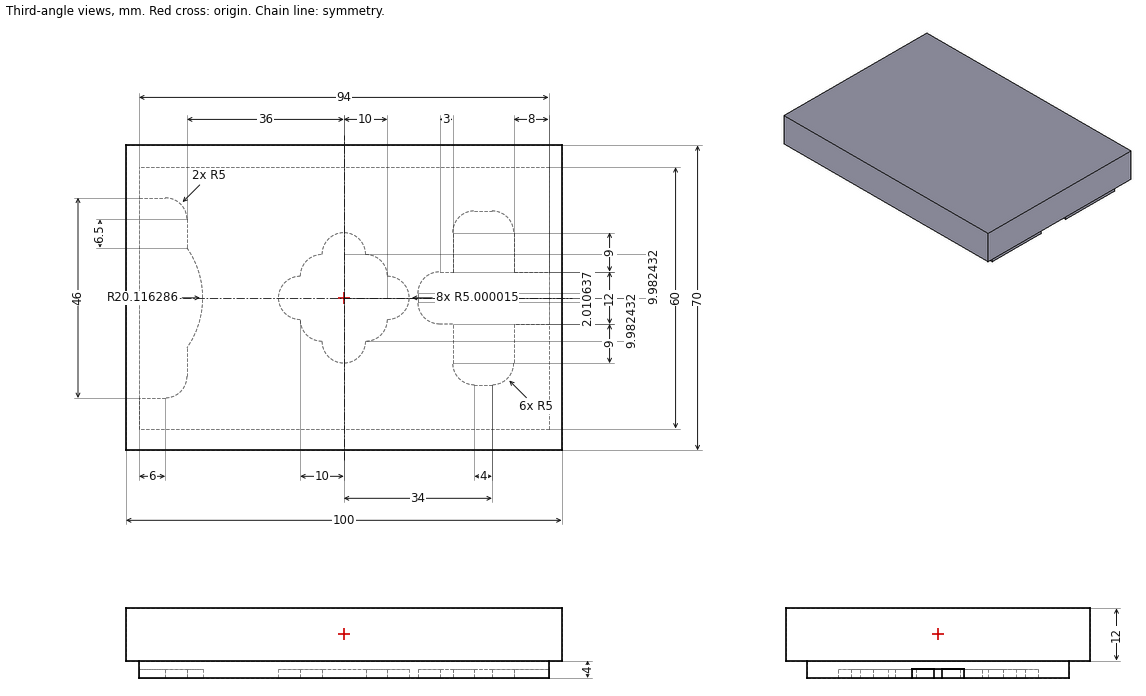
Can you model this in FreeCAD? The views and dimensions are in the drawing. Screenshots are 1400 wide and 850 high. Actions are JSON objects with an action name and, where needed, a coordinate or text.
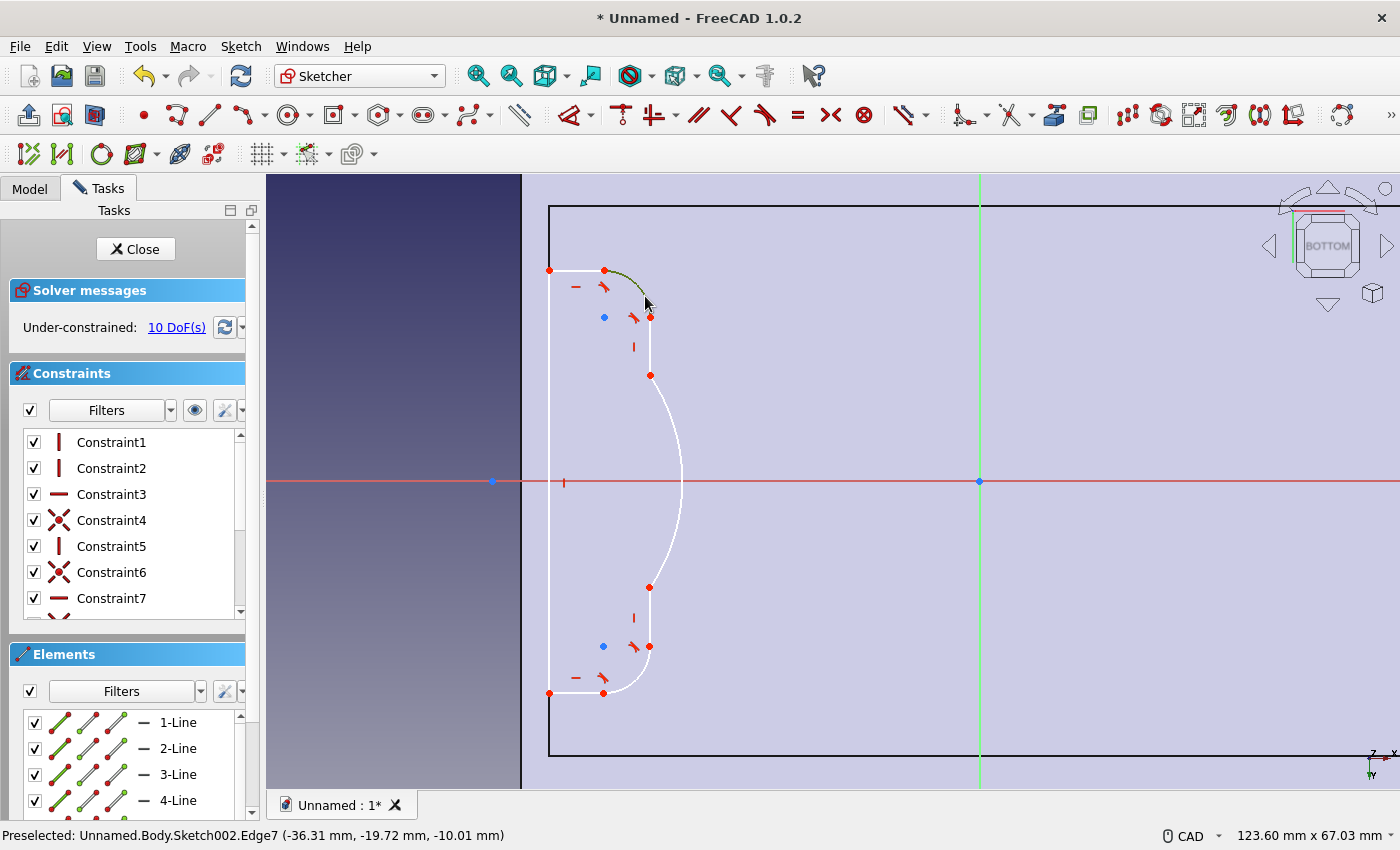
{"action": "left_click", "coordinate": [625, 688]}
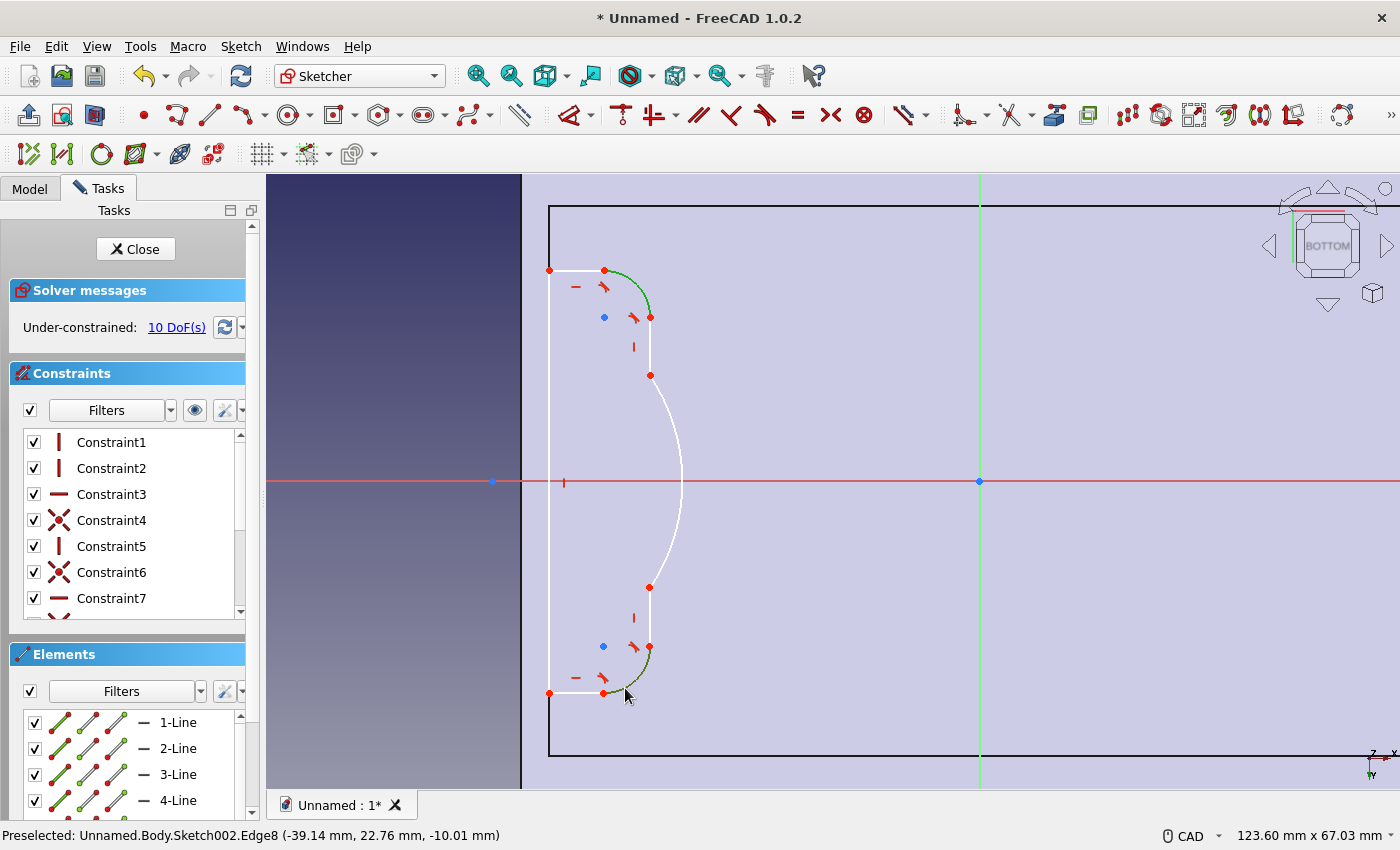
{"action": "left_click", "coordinate": [798, 116]}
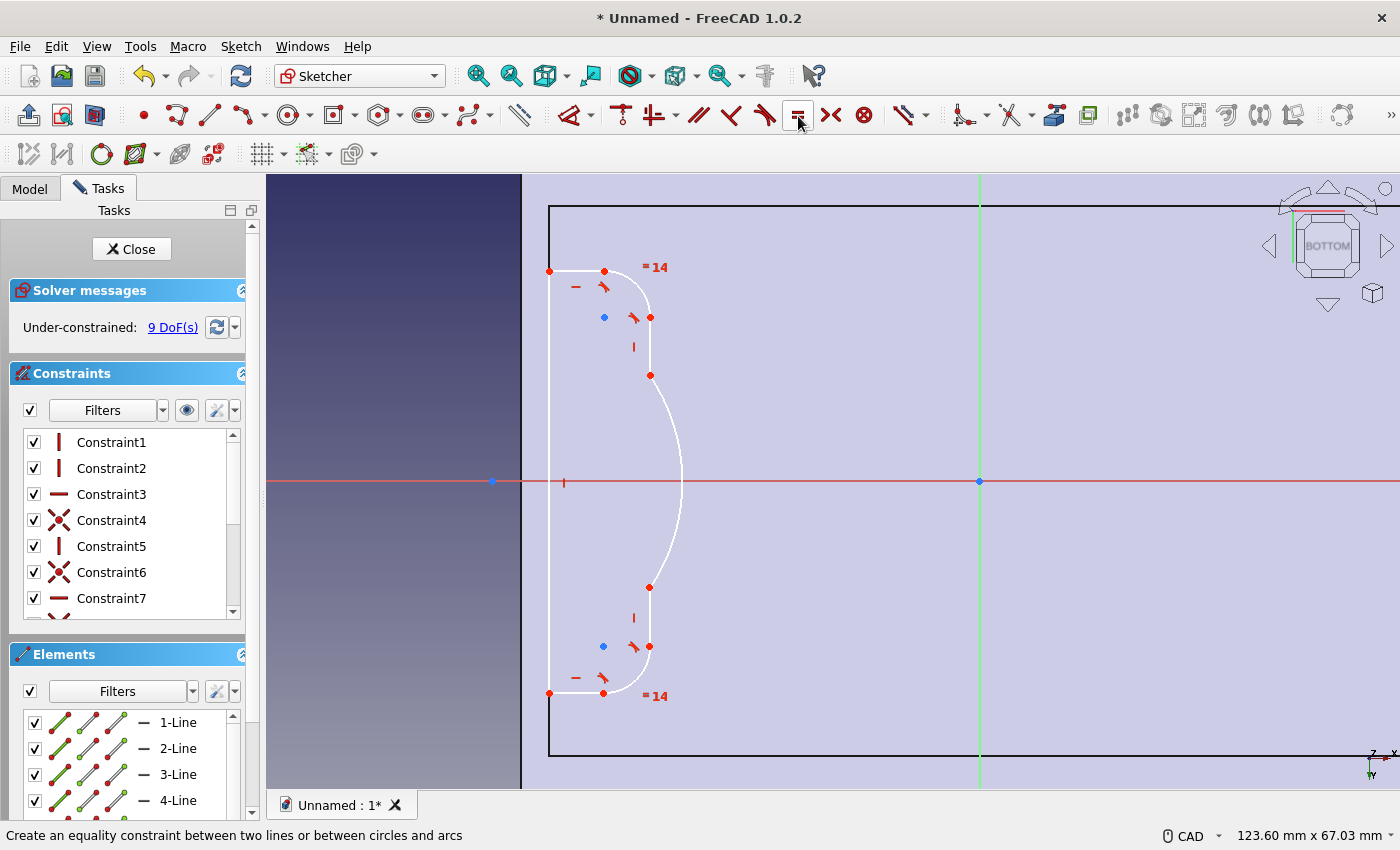
{"action": "left_click", "coordinate": [492, 482]}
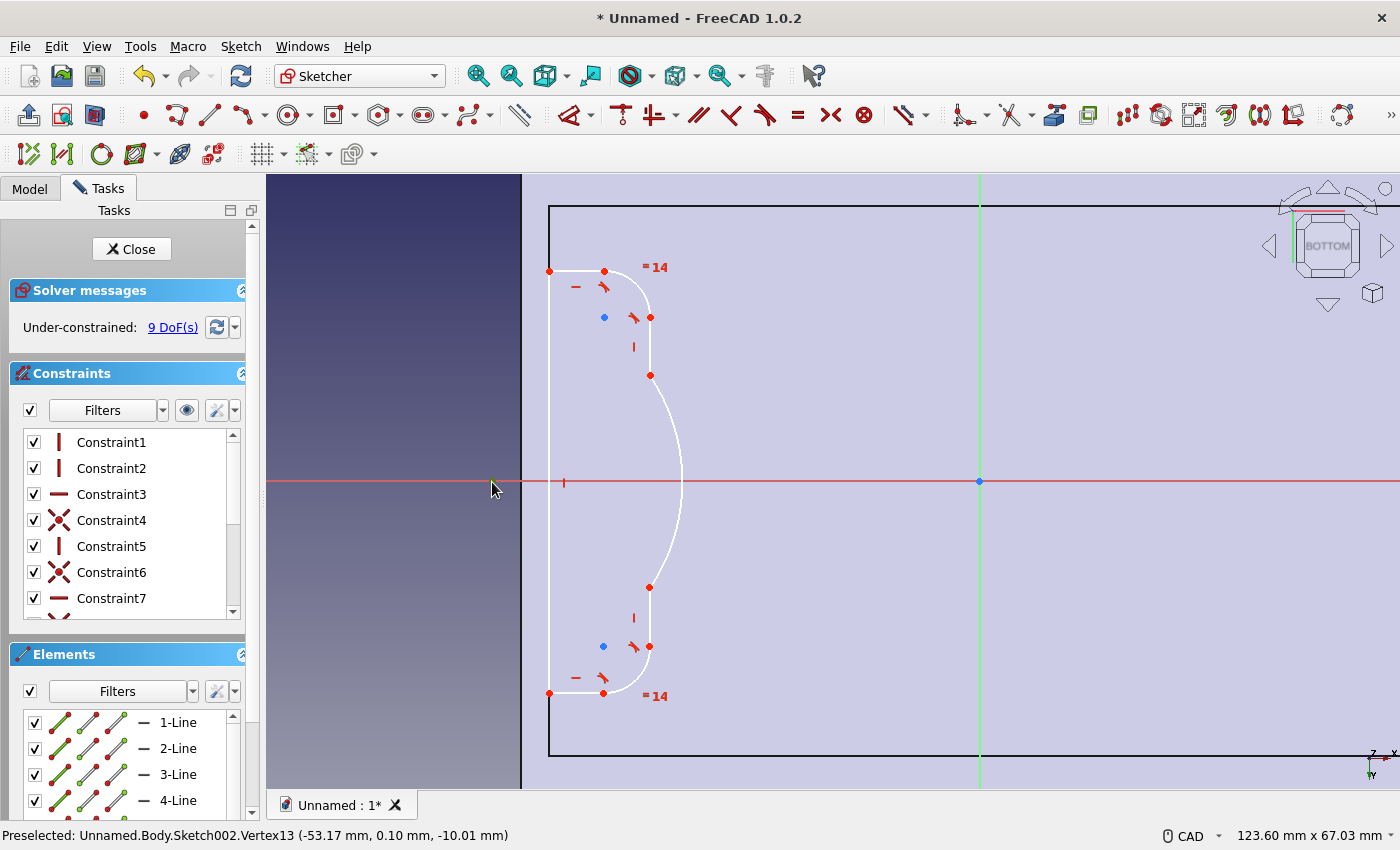
{"action": "left_click", "coordinate": [361, 481]}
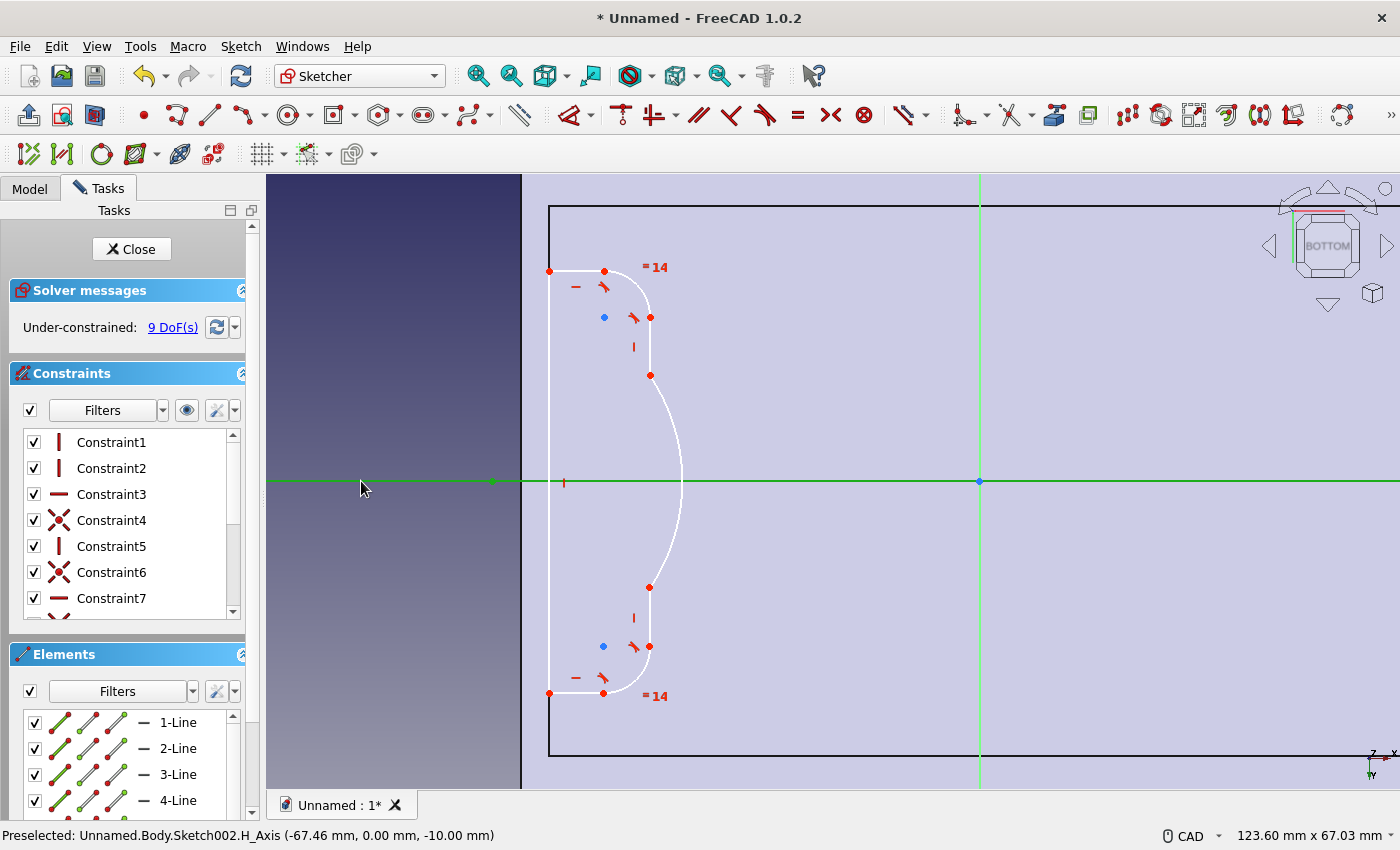
{"action": "left_click", "coordinate": [621, 116]}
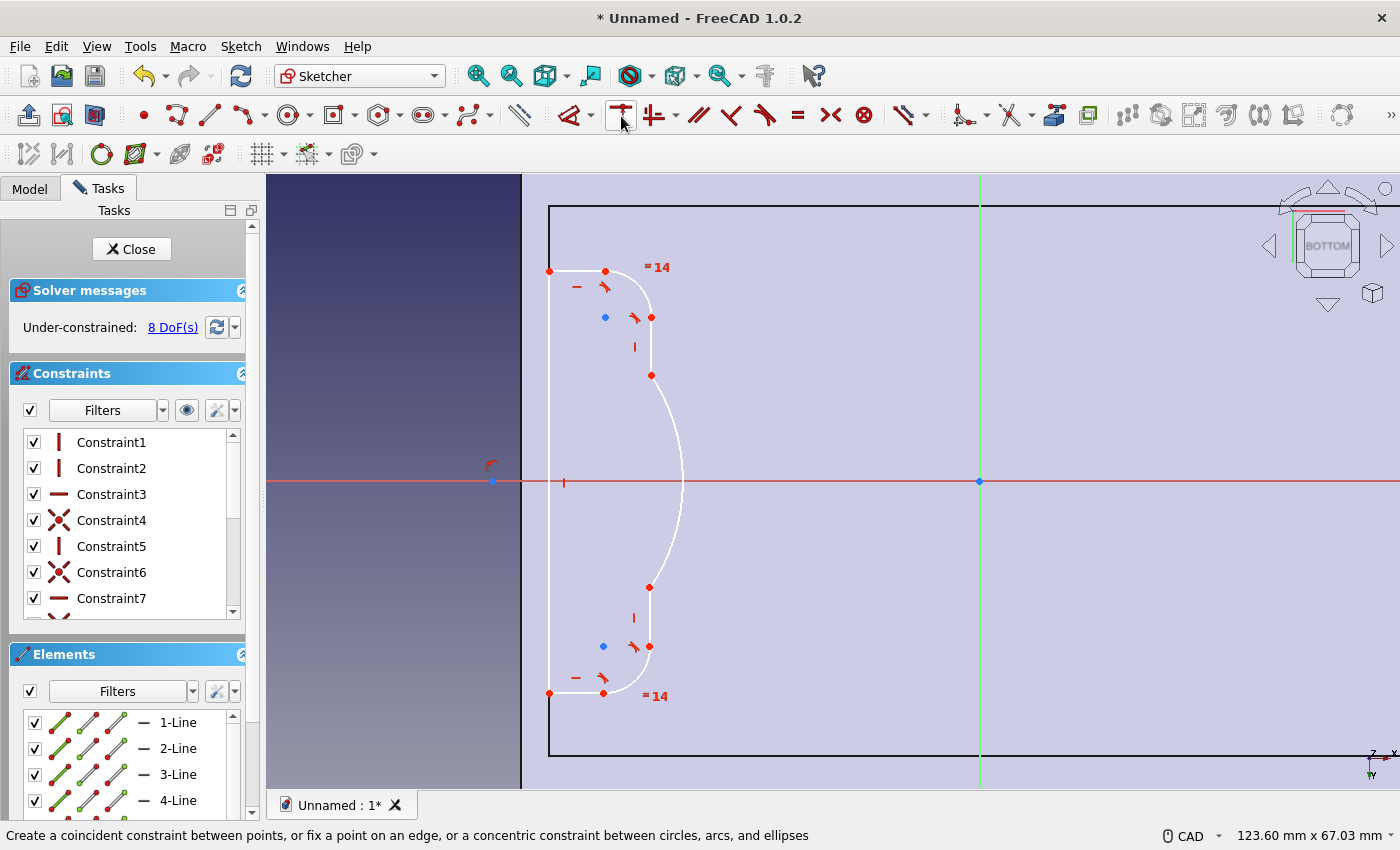
{"action": "left_click", "coordinate": [605, 317]}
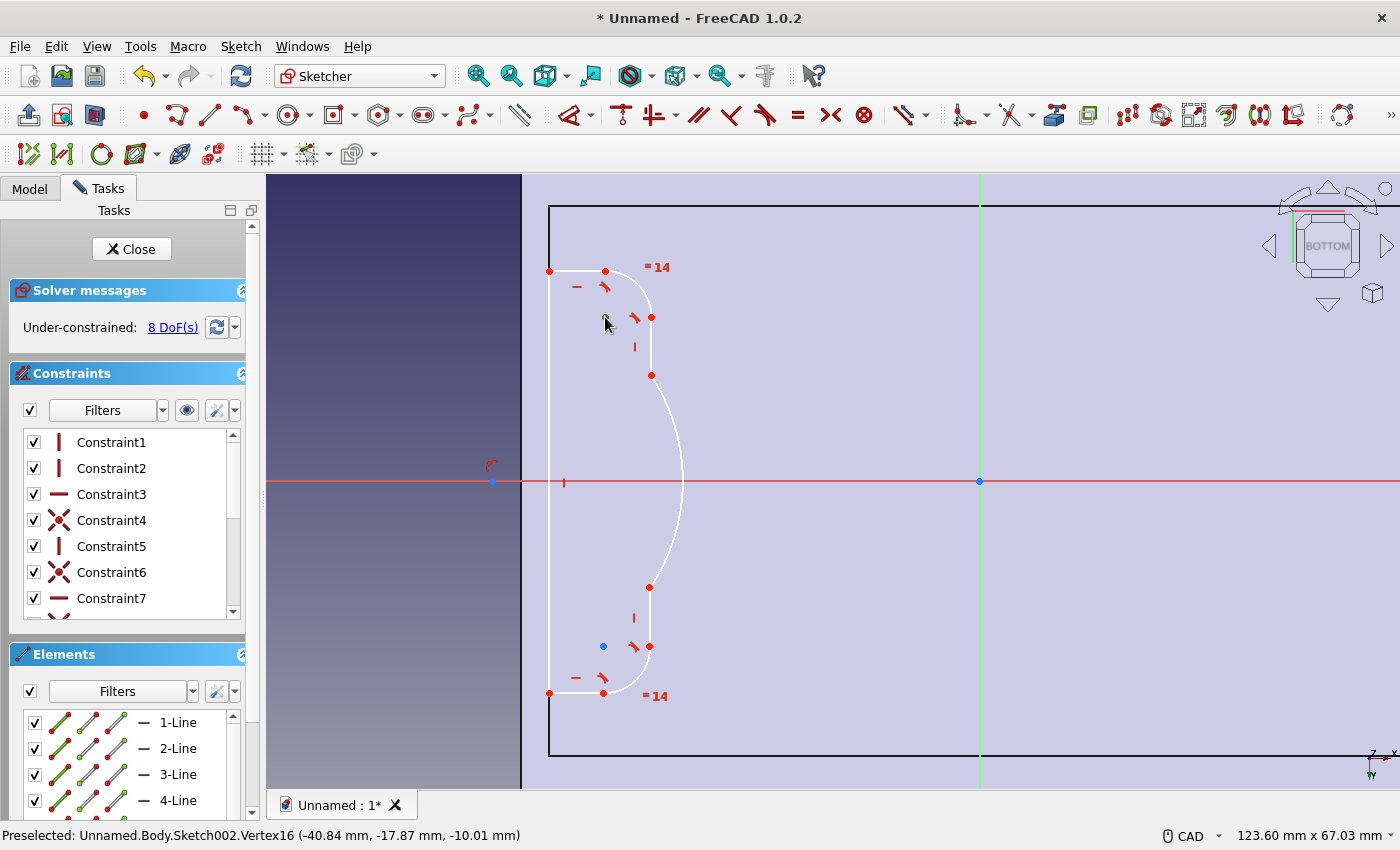
{"action": "left_click", "coordinate": [604, 647]}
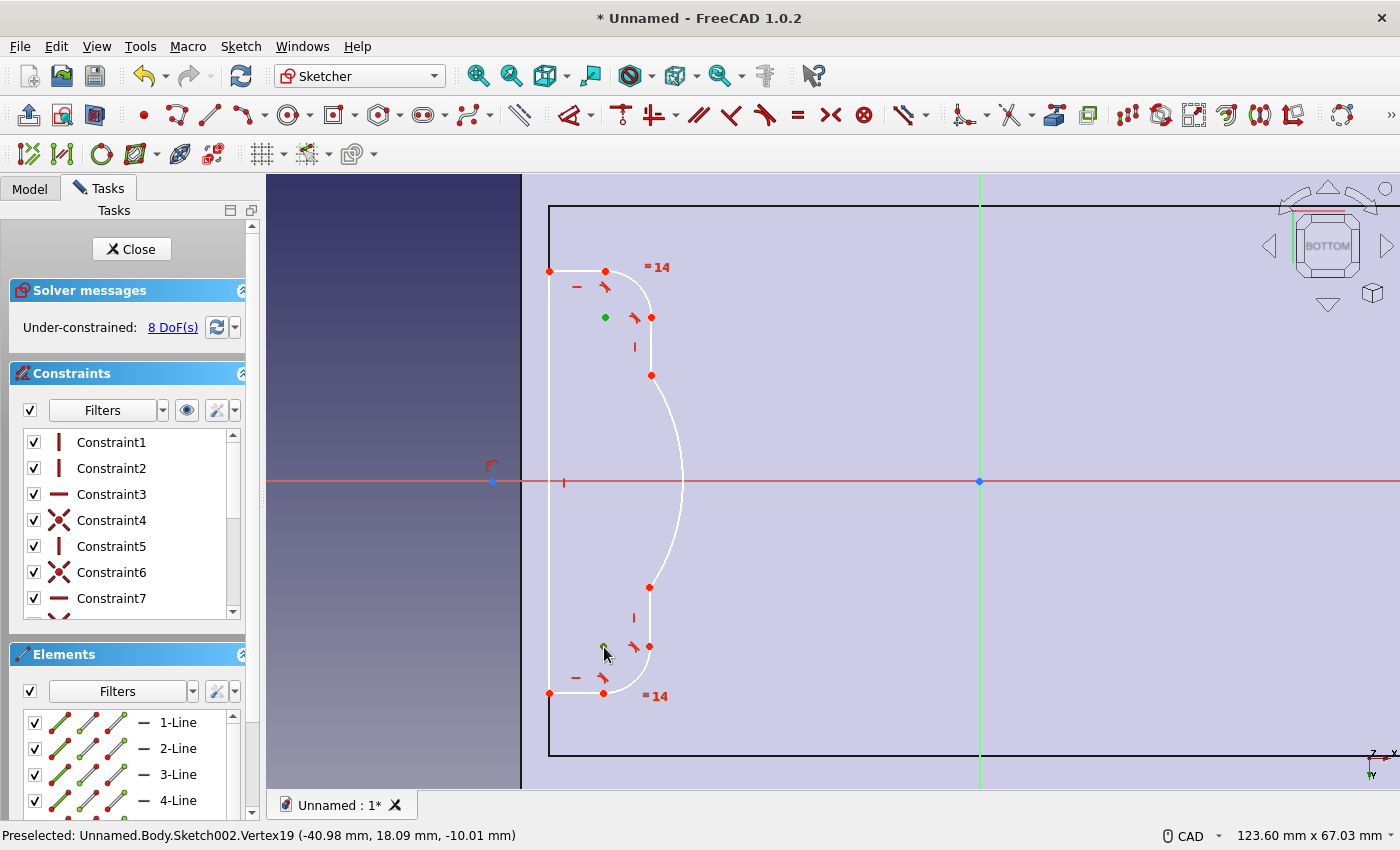
{"action": "left_click", "coordinate": [361, 481]}